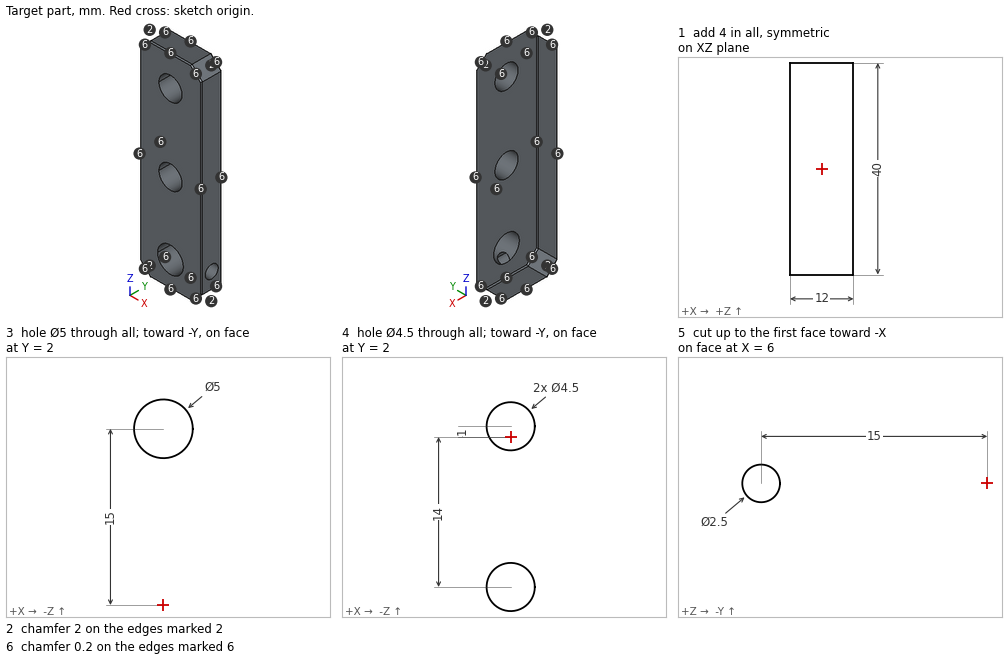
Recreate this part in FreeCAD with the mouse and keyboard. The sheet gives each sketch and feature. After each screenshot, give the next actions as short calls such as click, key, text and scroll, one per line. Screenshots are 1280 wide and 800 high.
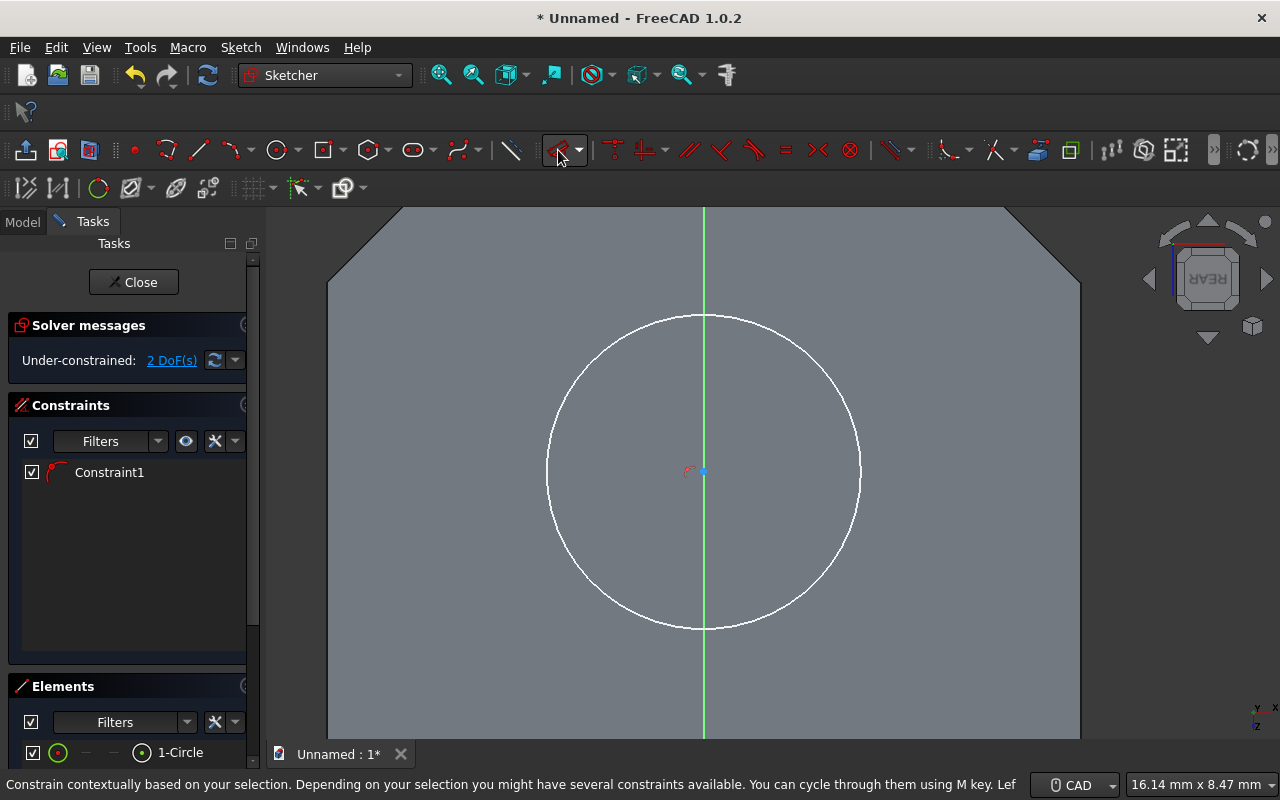
click(815, 361)
click(838, 338)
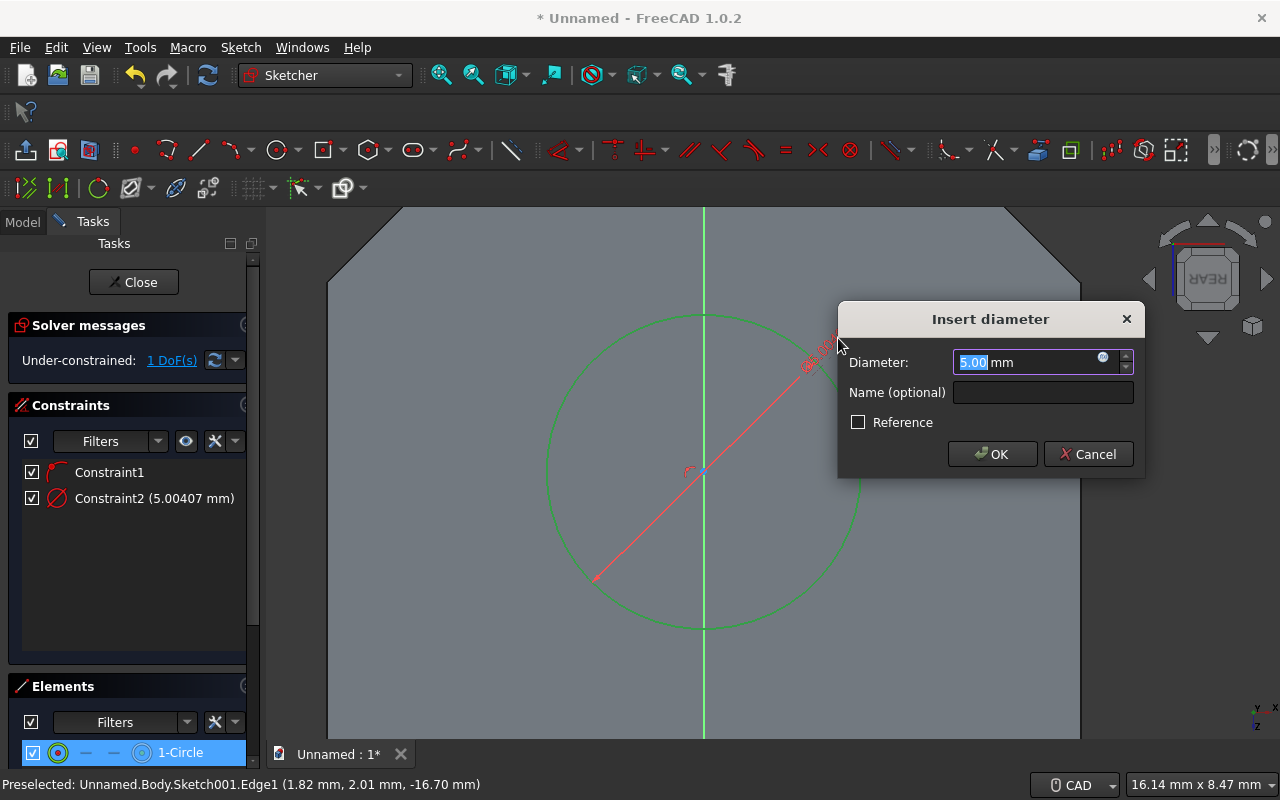
text(5)
key(Return)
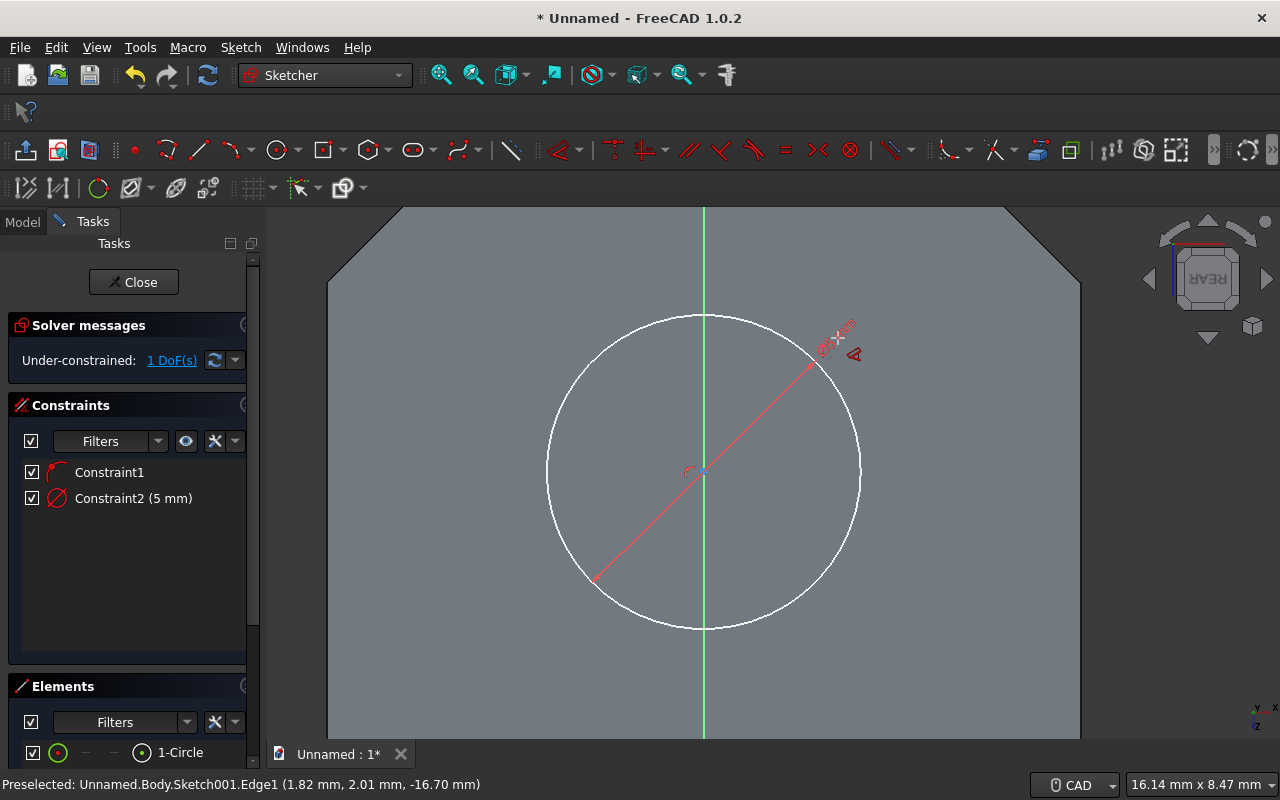
click(704, 472)
click(738, 592)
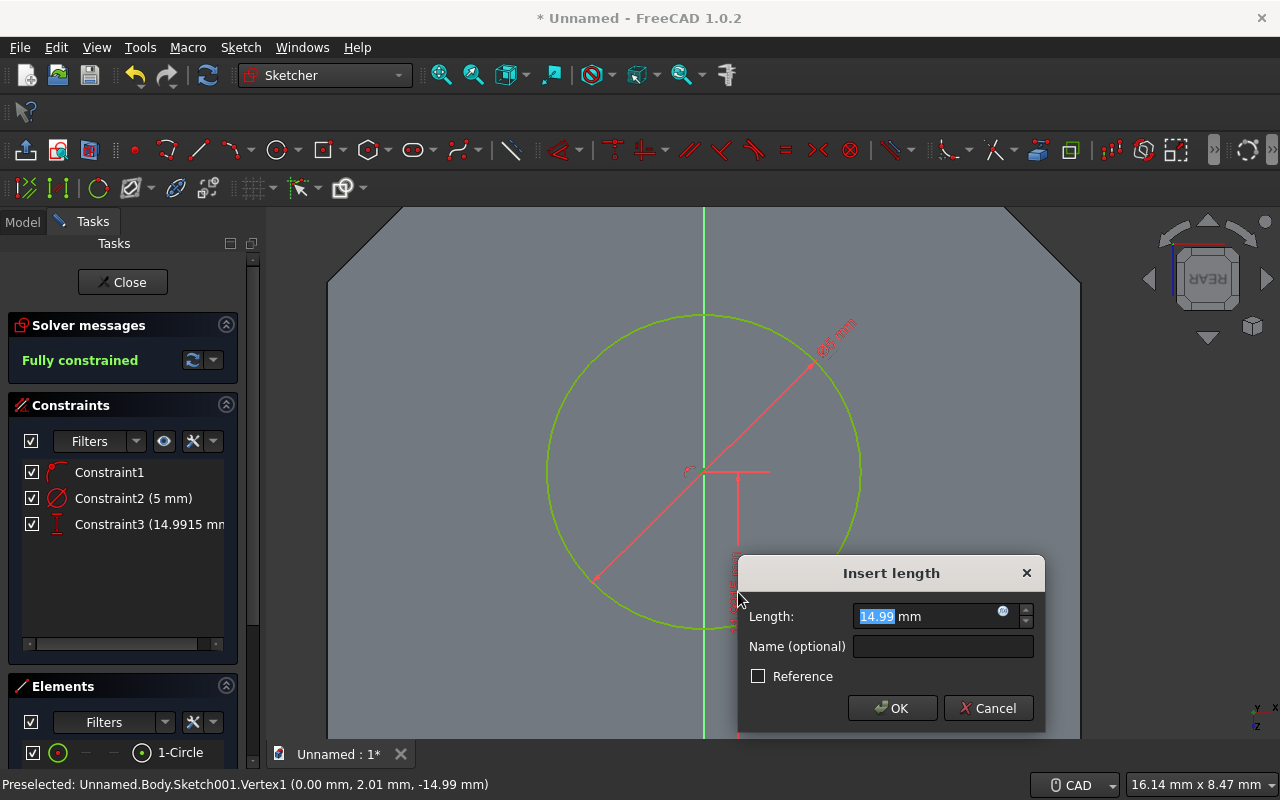
text(15)
key(Return)
key(Escape)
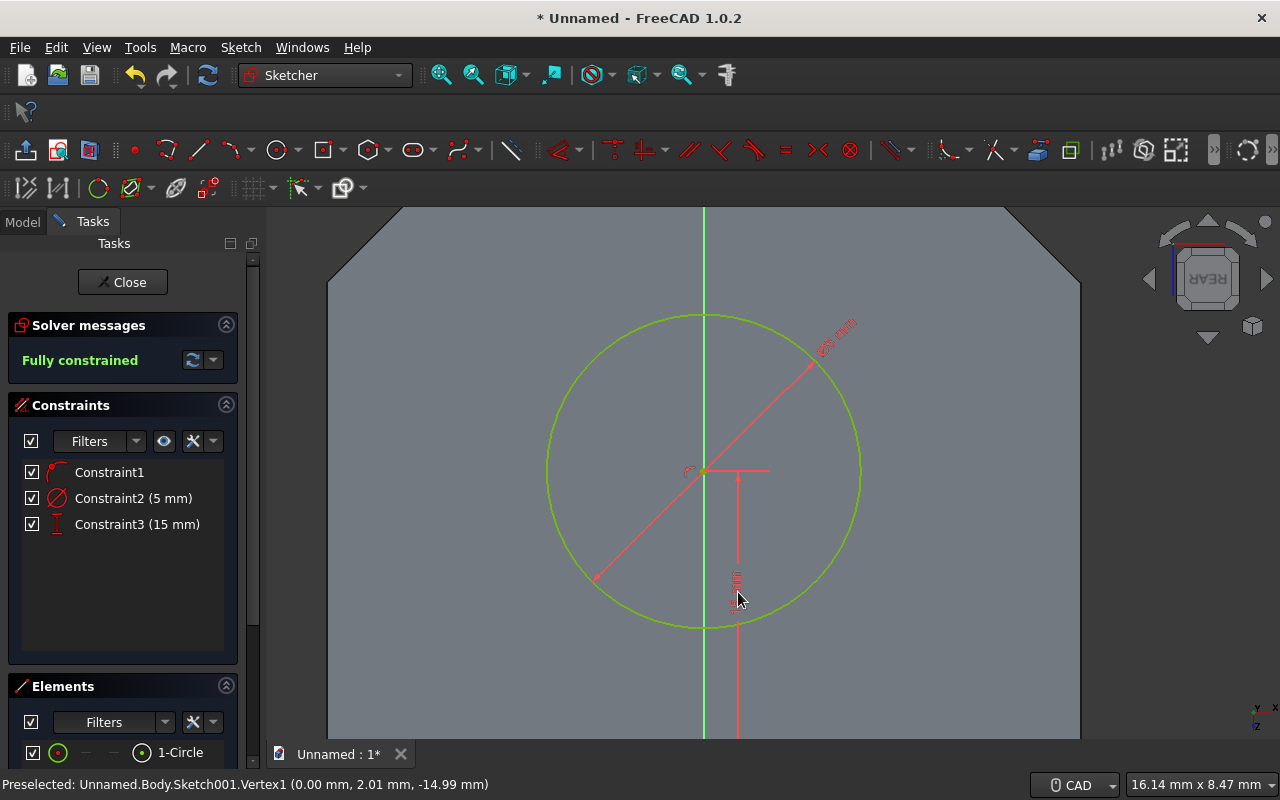
click(123, 282)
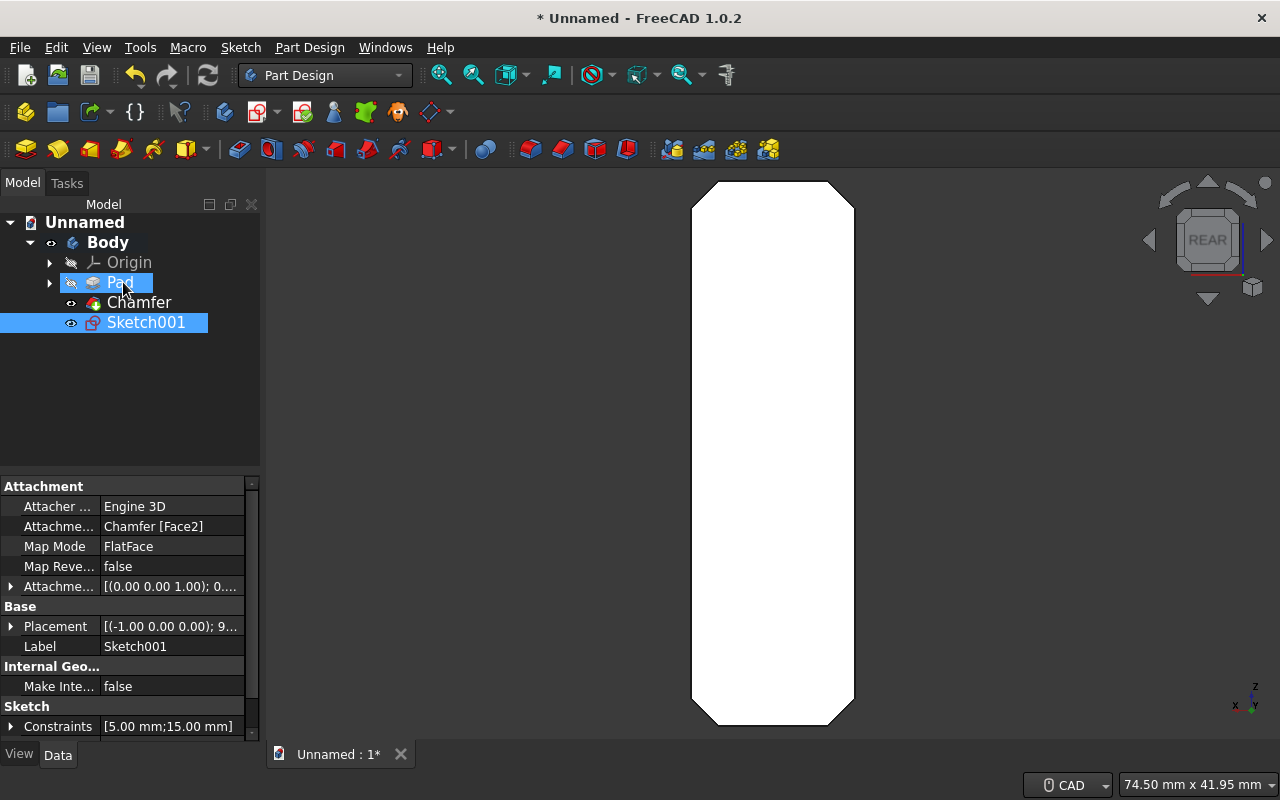
click(272, 150)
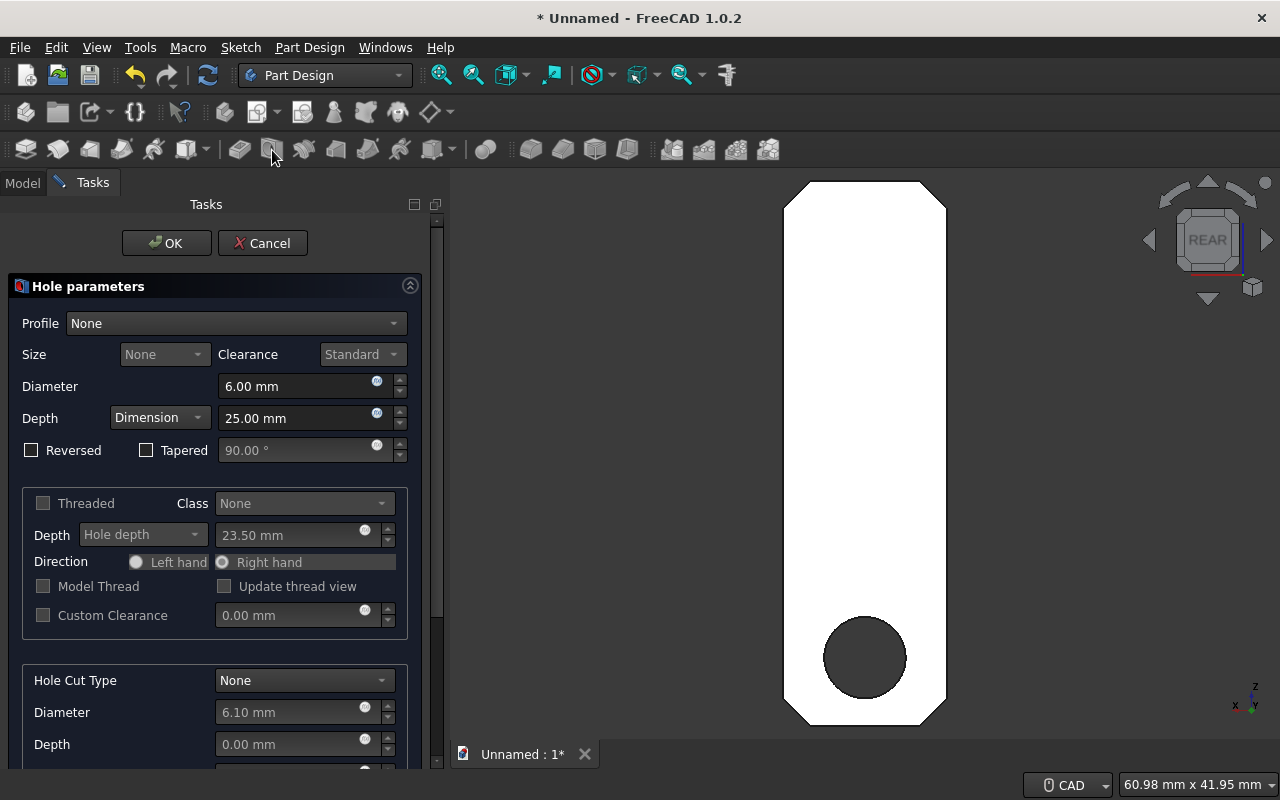
triple_click(305, 386)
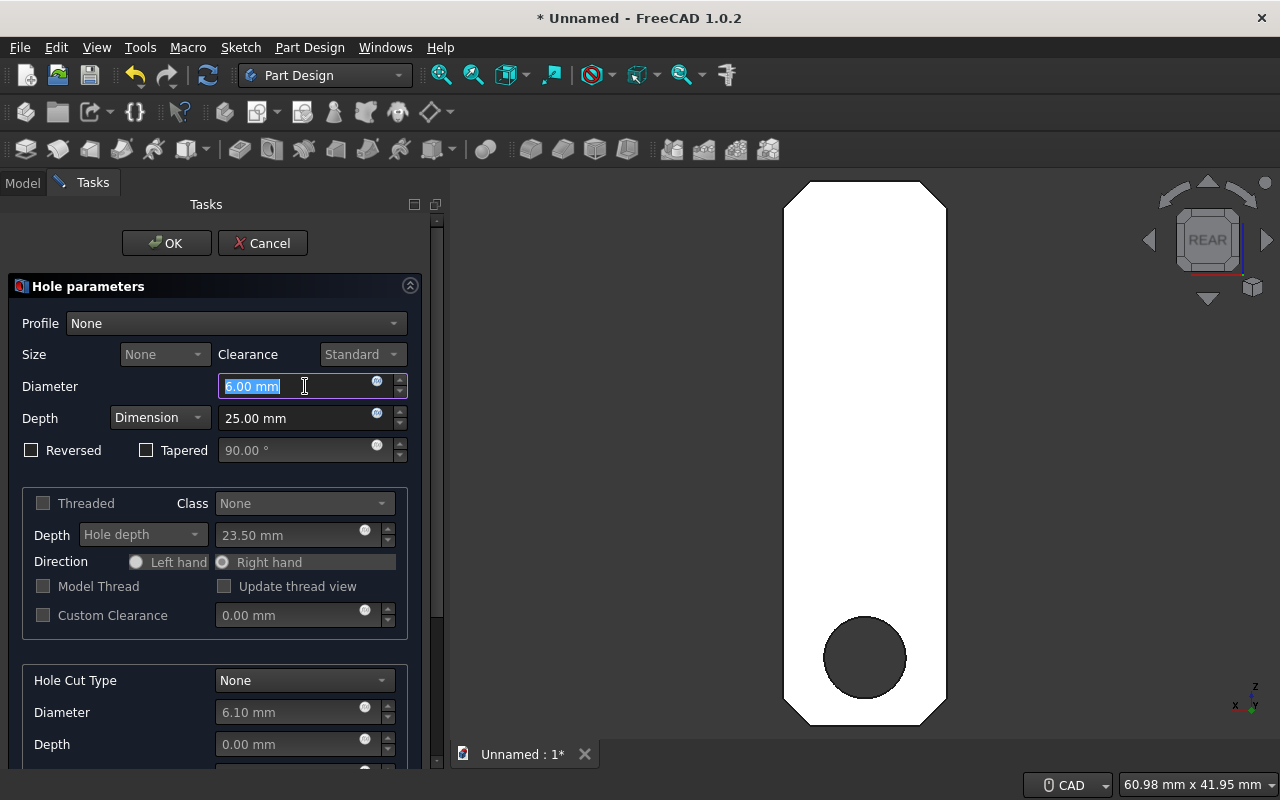
text(5)
key(Tab)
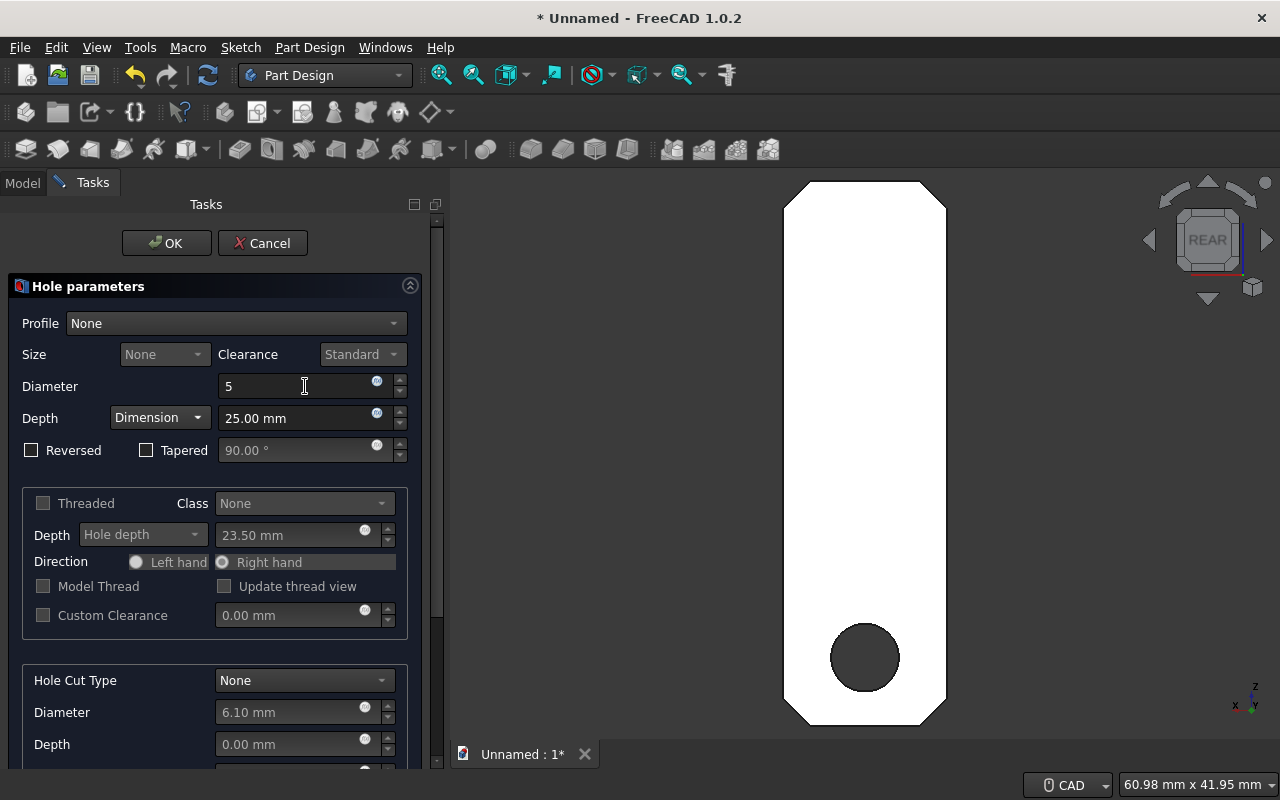
click(161, 418)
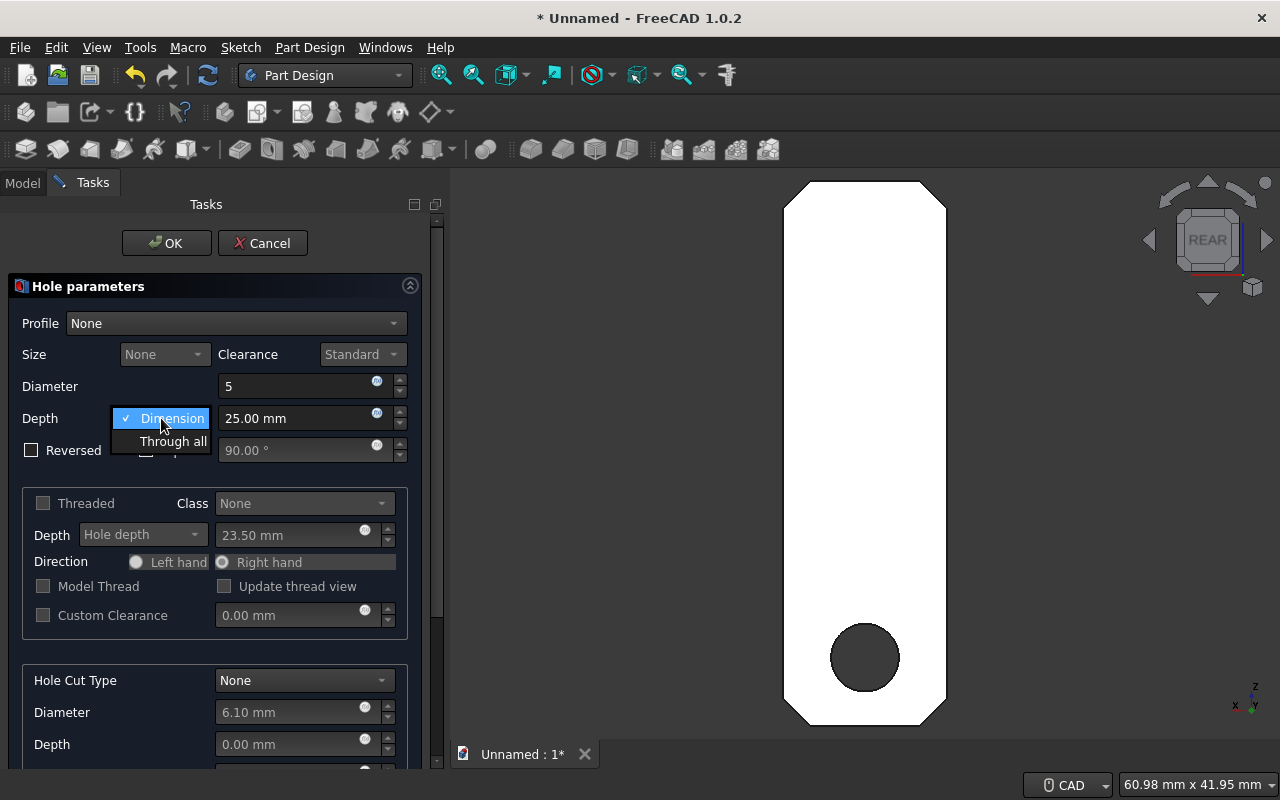
click(160, 442)